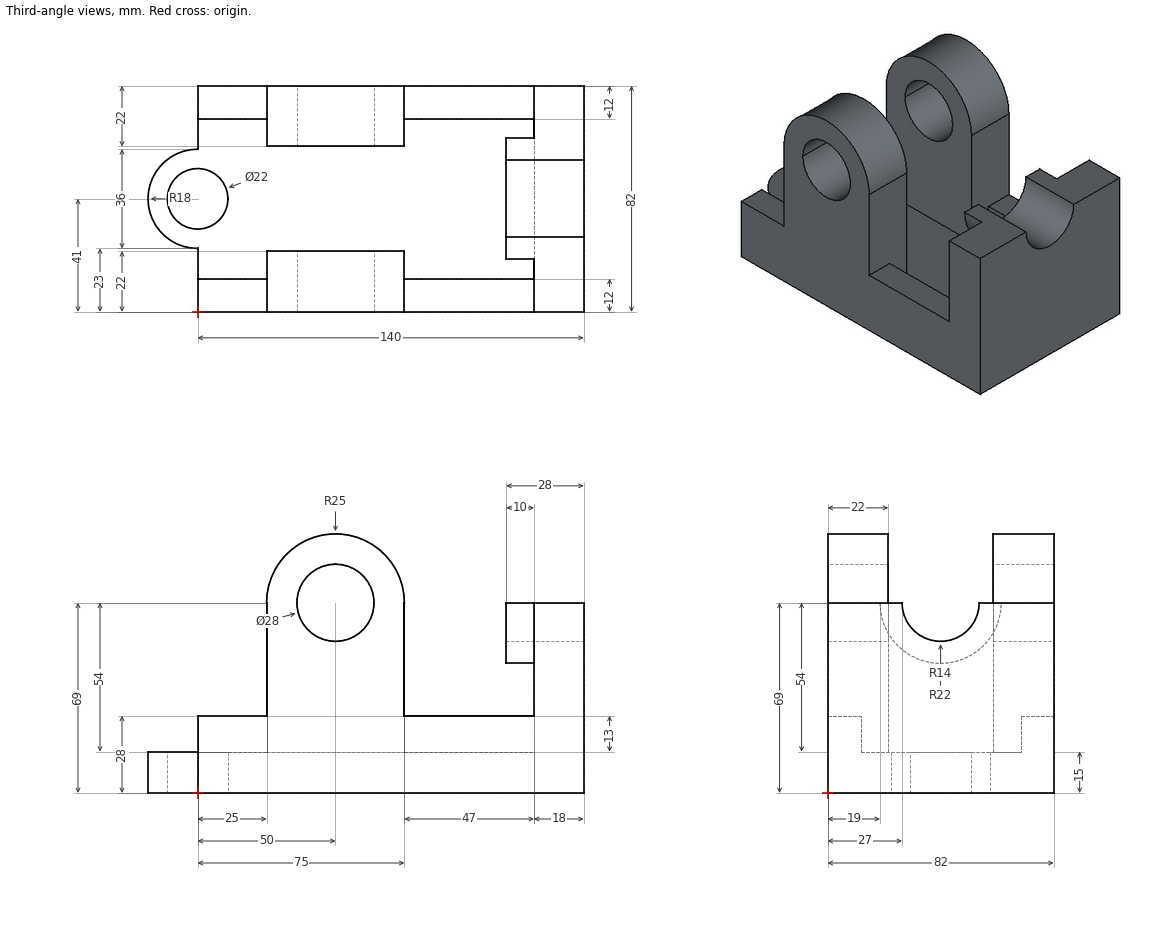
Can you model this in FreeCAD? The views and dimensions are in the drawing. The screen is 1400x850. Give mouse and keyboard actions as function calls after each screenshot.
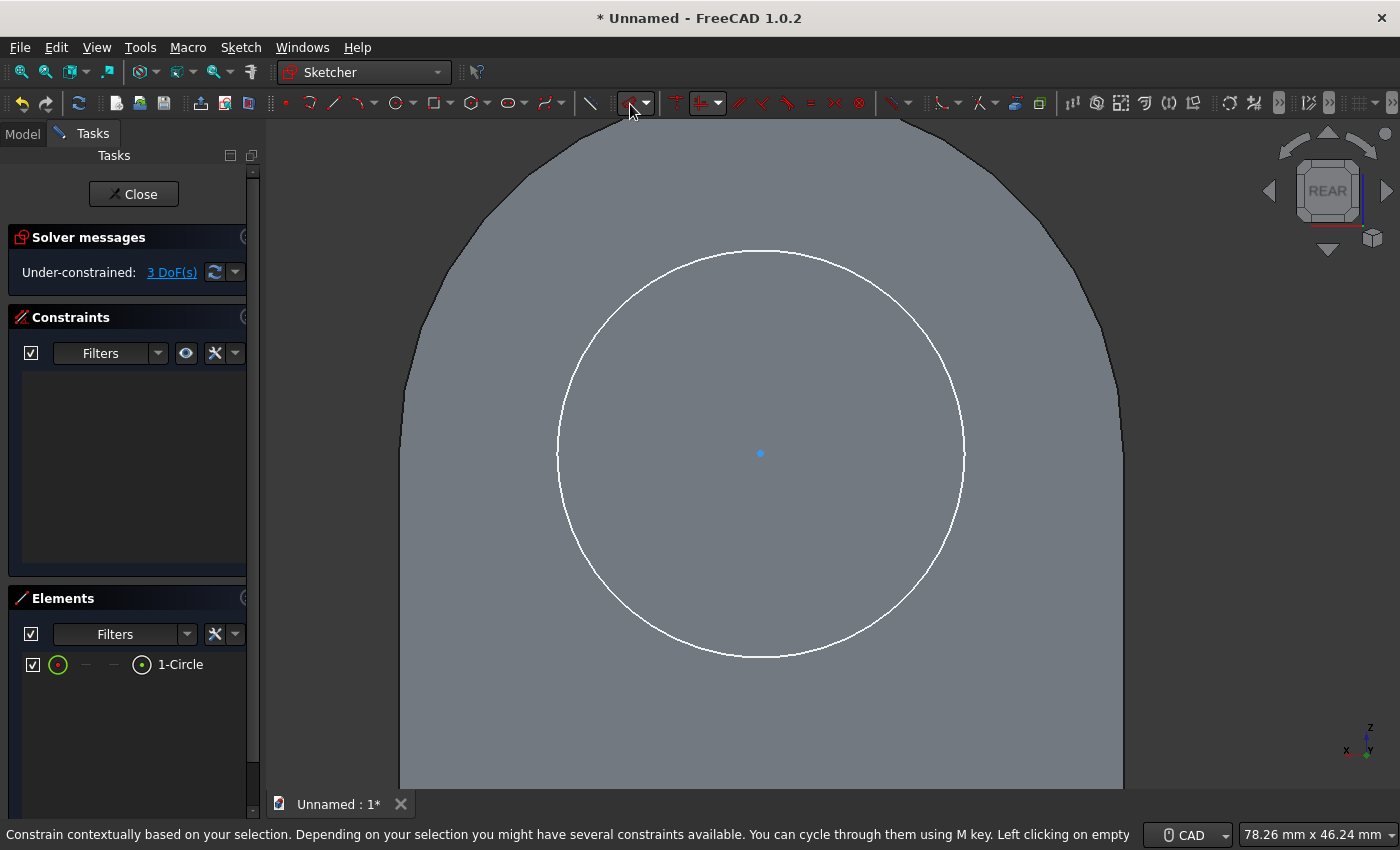
click(905, 310)
click(928, 287)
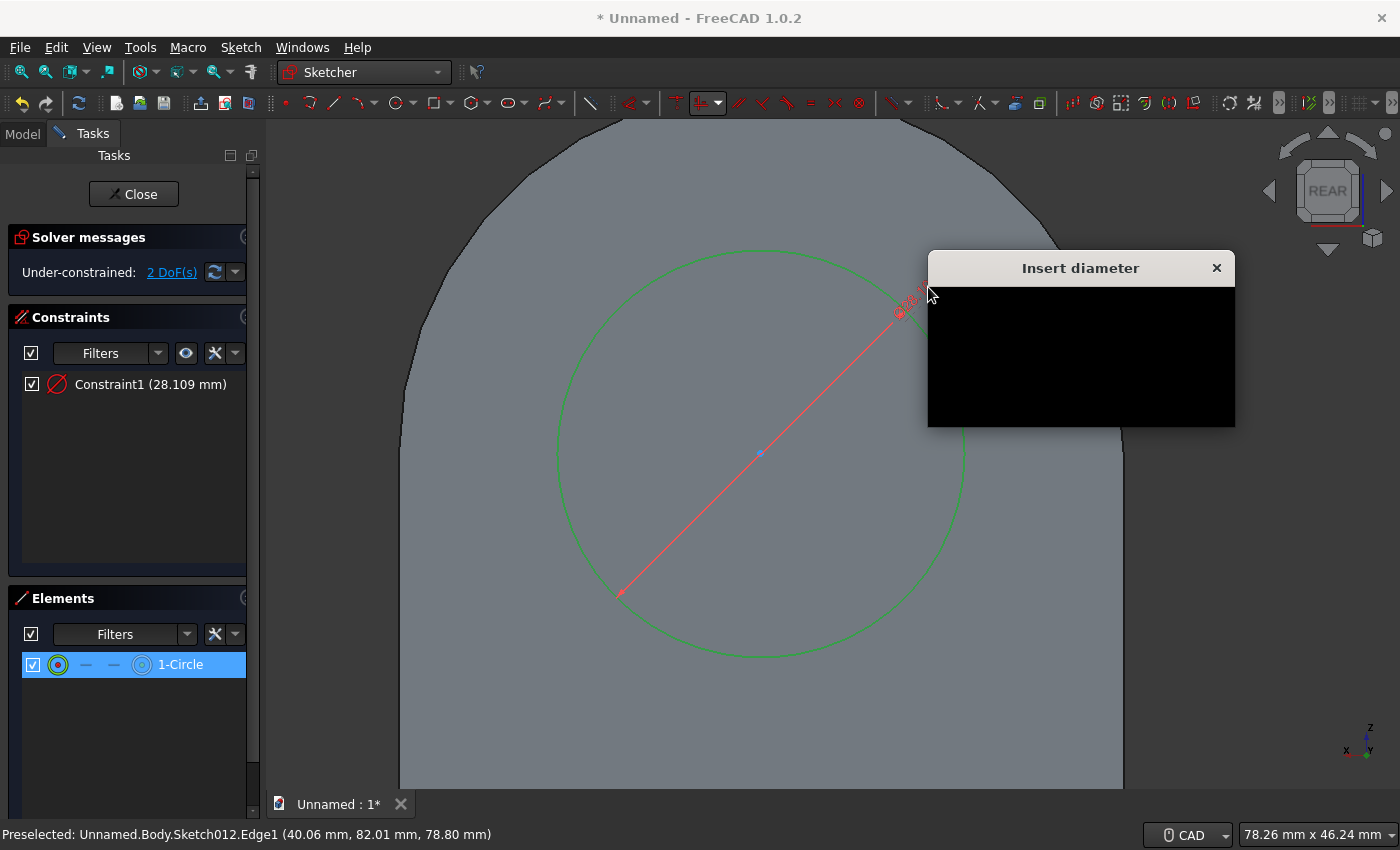
text(28)
key(Return)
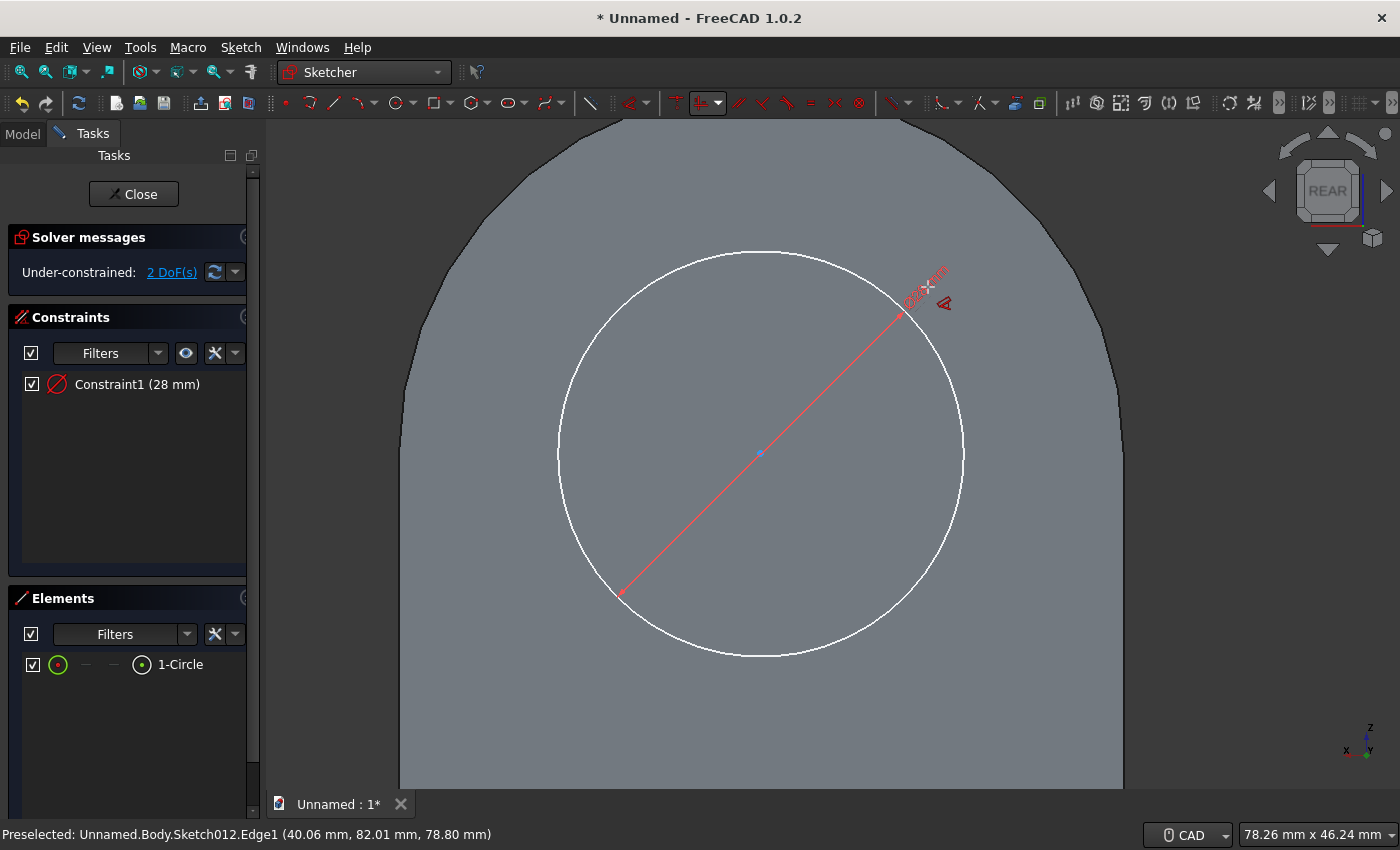
click(761, 454)
click(998, 420)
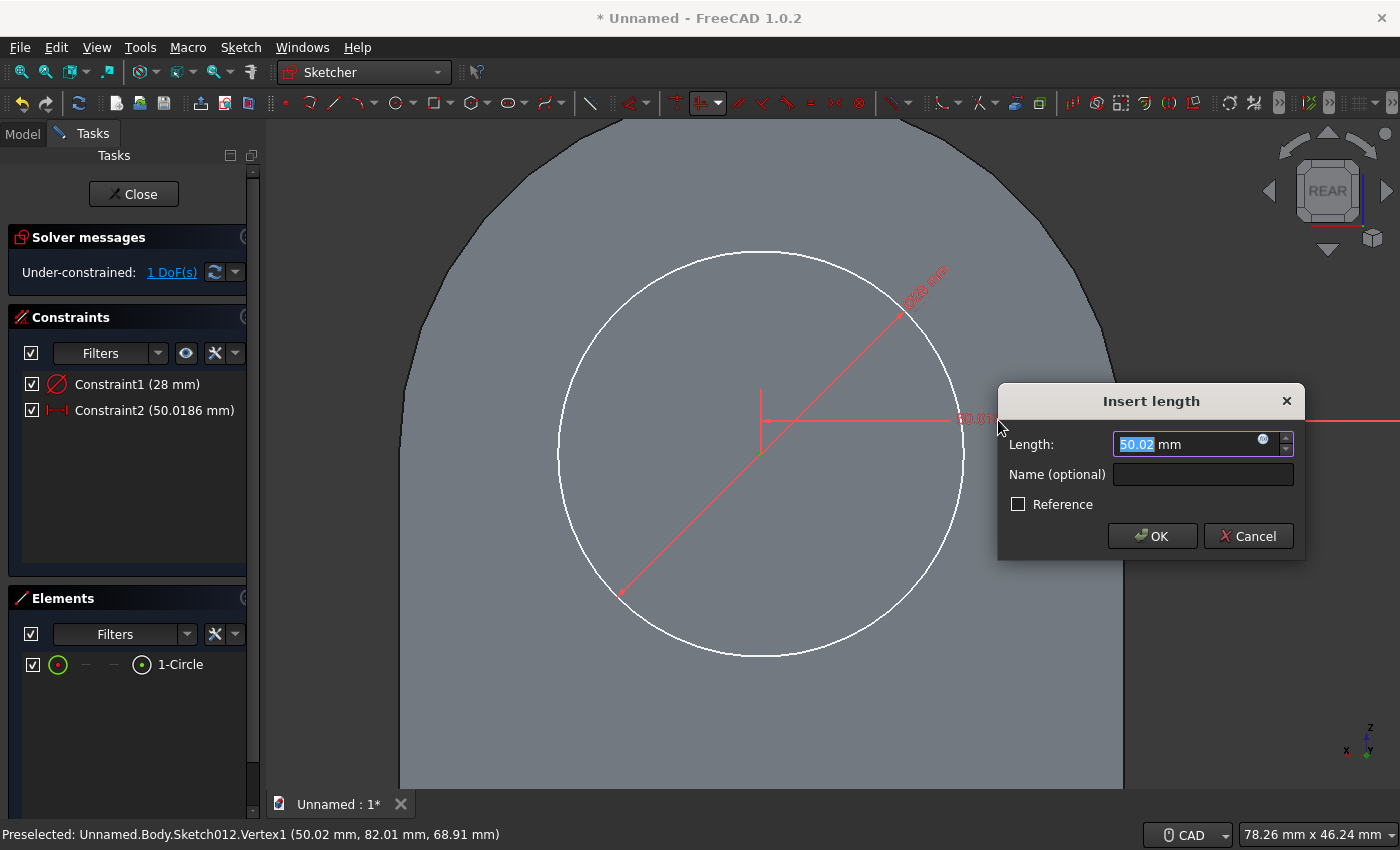
text(50)
key(Return)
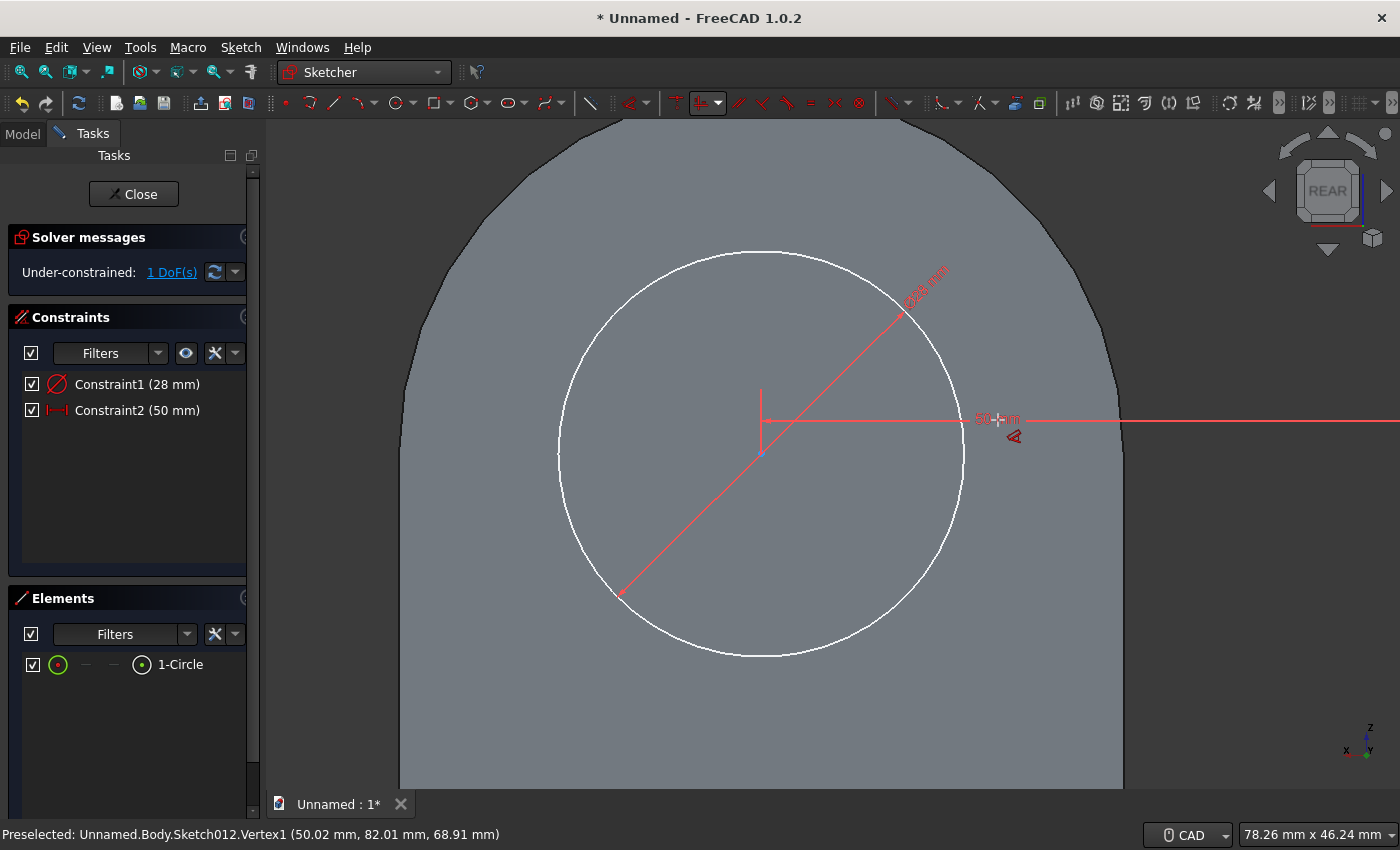
click(761, 454)
click(727, 608)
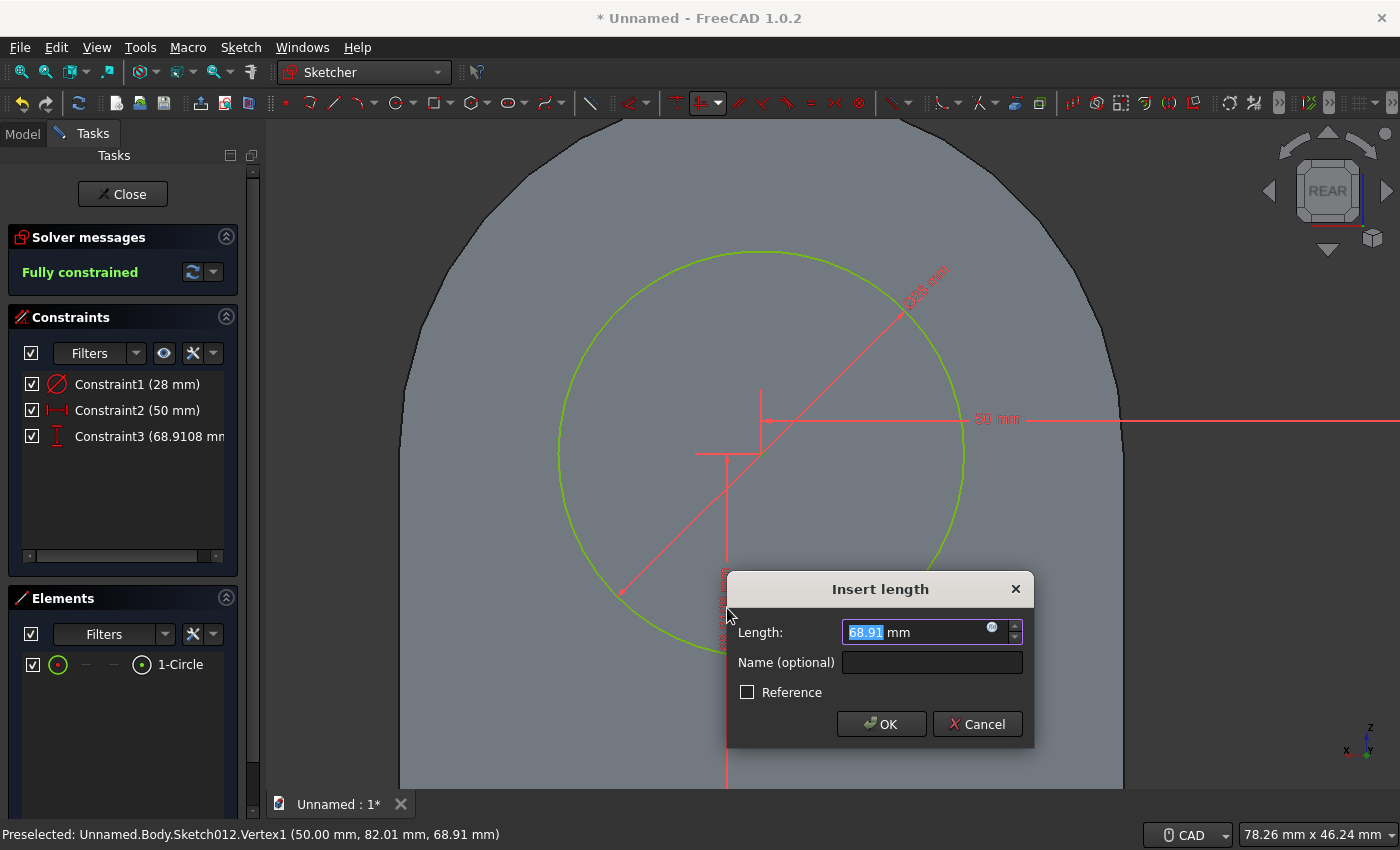
text(69)
key(Return)
key(Escape)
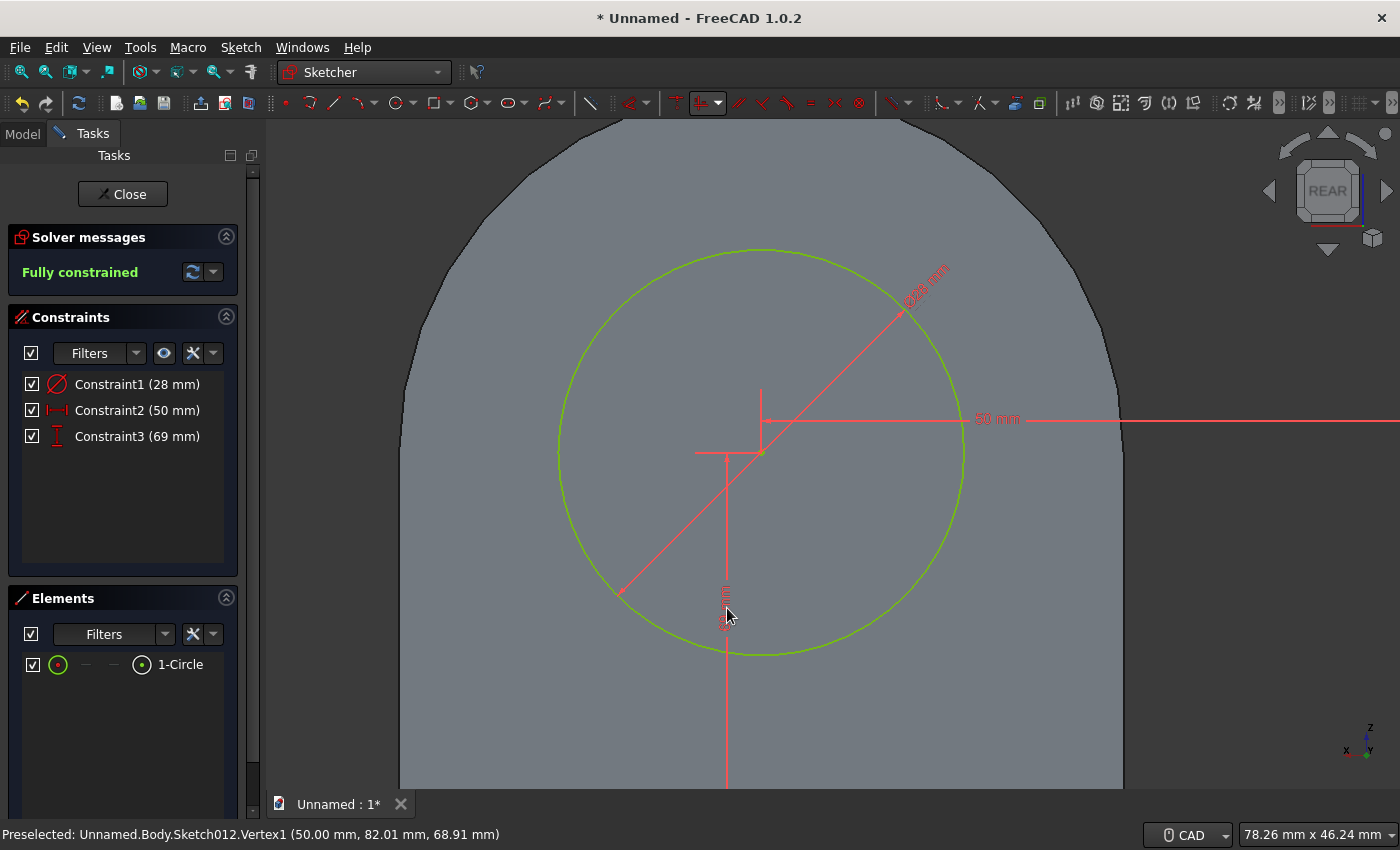
click(123, 194)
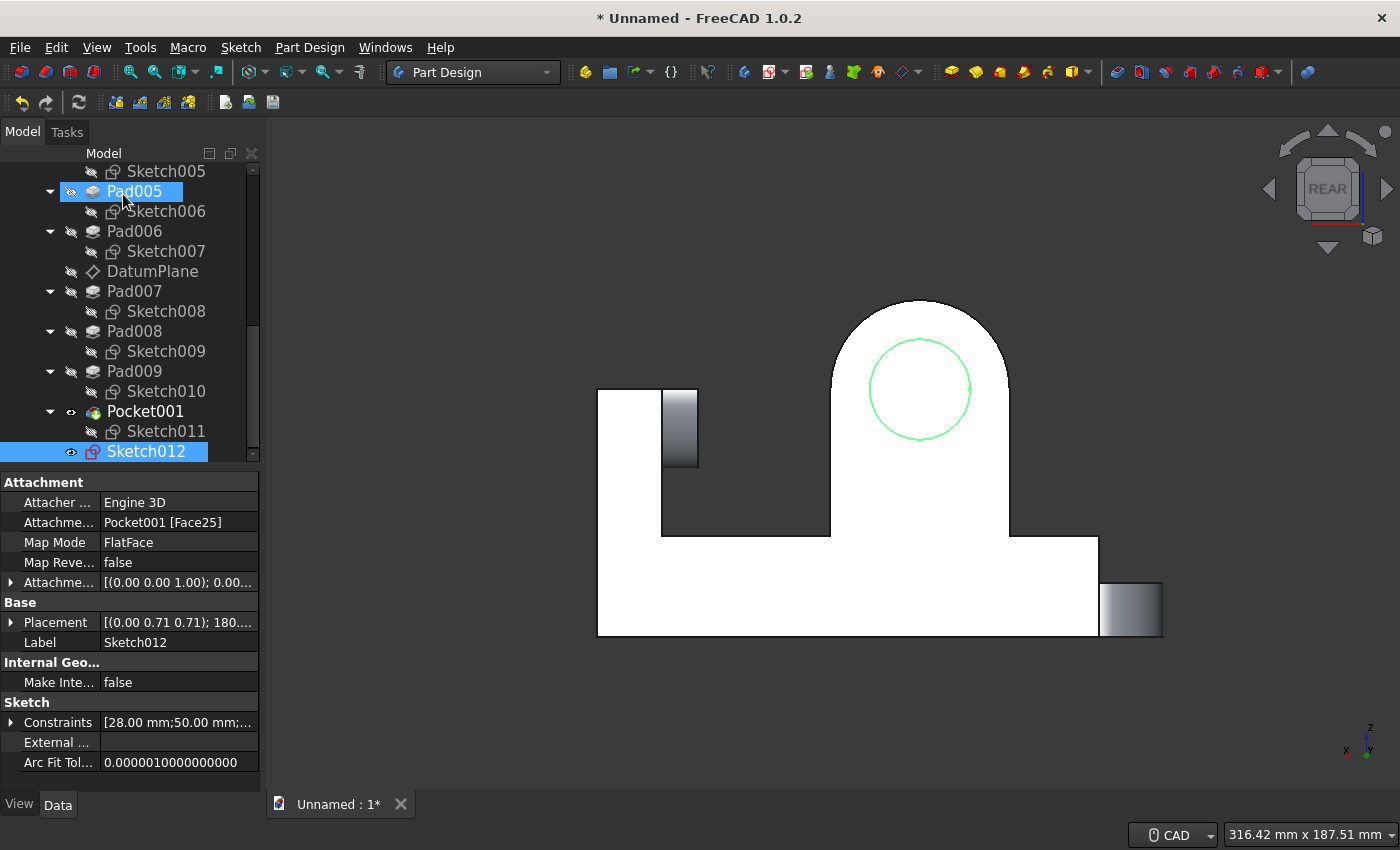
click(1118, 72)